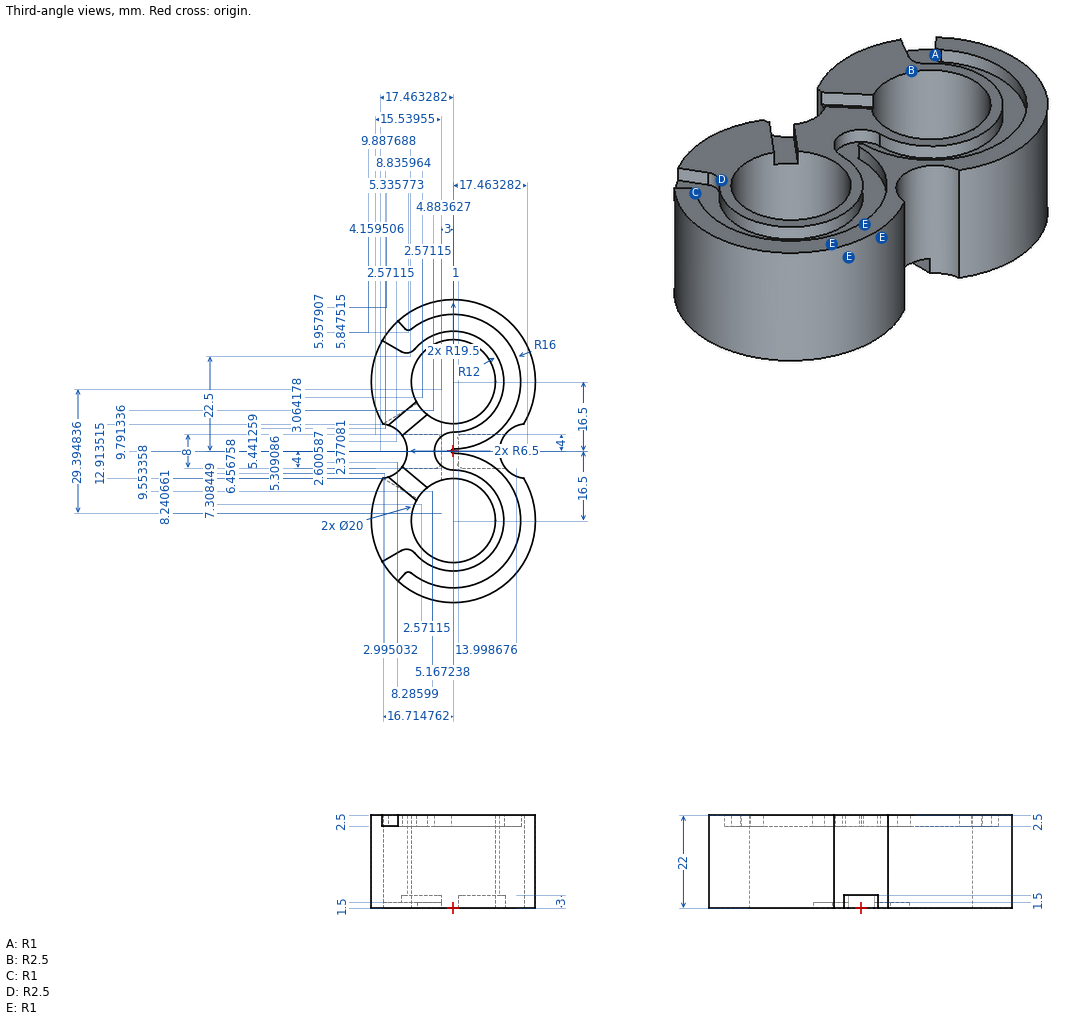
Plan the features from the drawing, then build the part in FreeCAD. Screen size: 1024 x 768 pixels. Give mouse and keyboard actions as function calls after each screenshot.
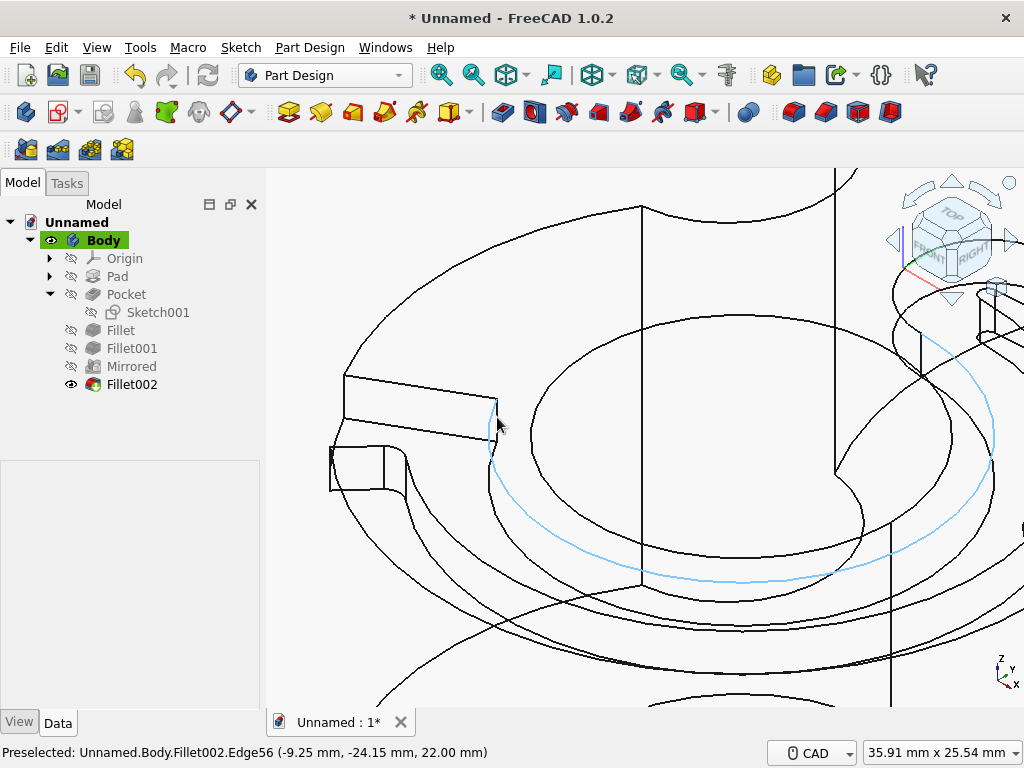
click(497, 419)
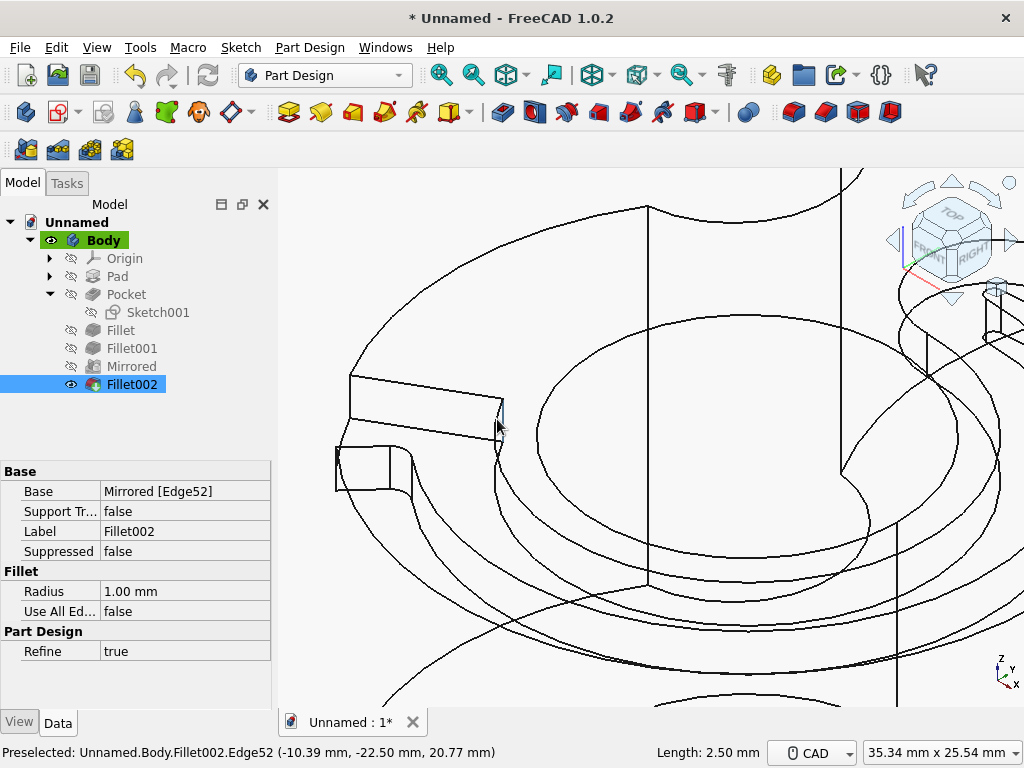
key(v)
key(1)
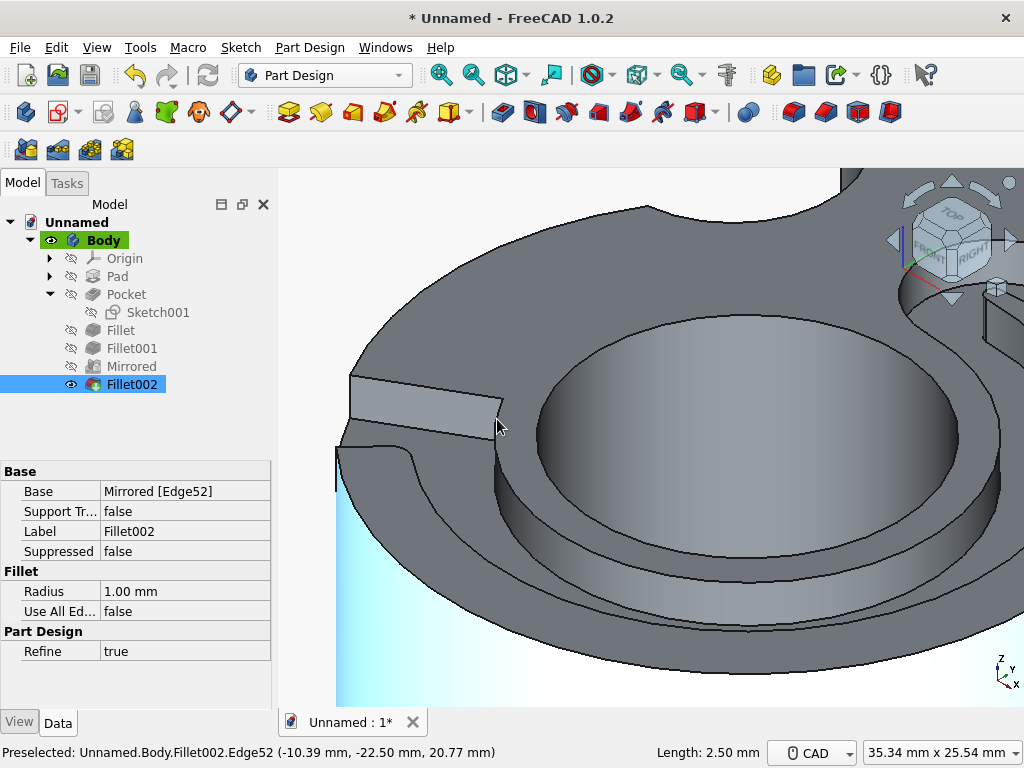
click(794, 112)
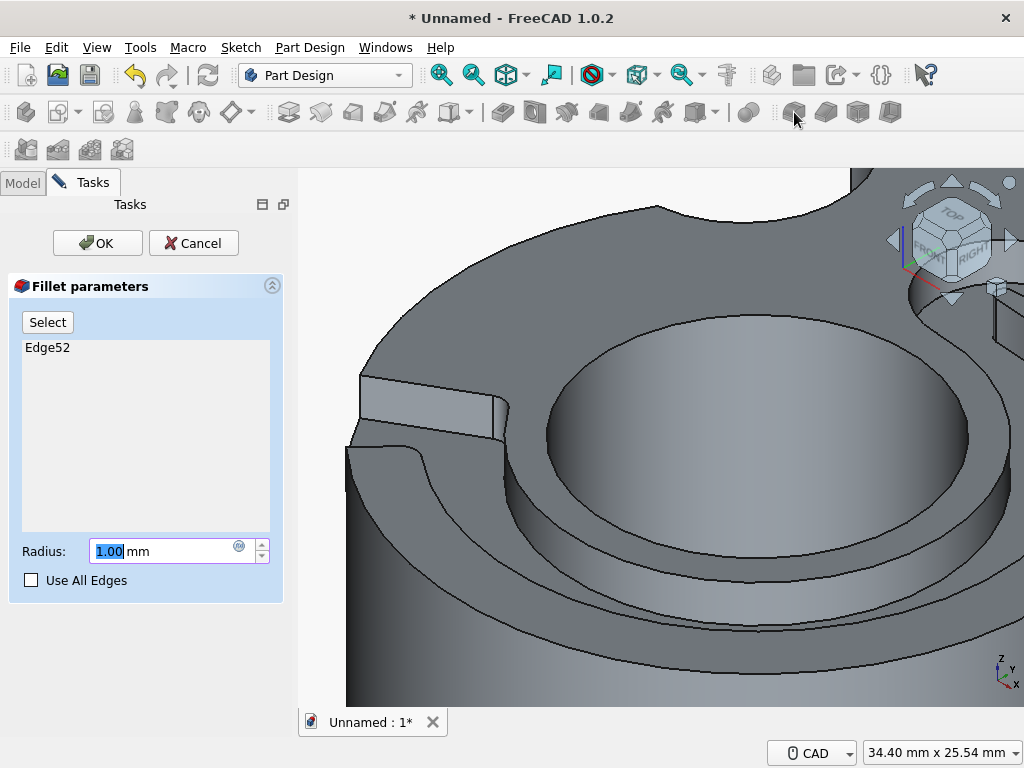
text(2.5)
key(Tab)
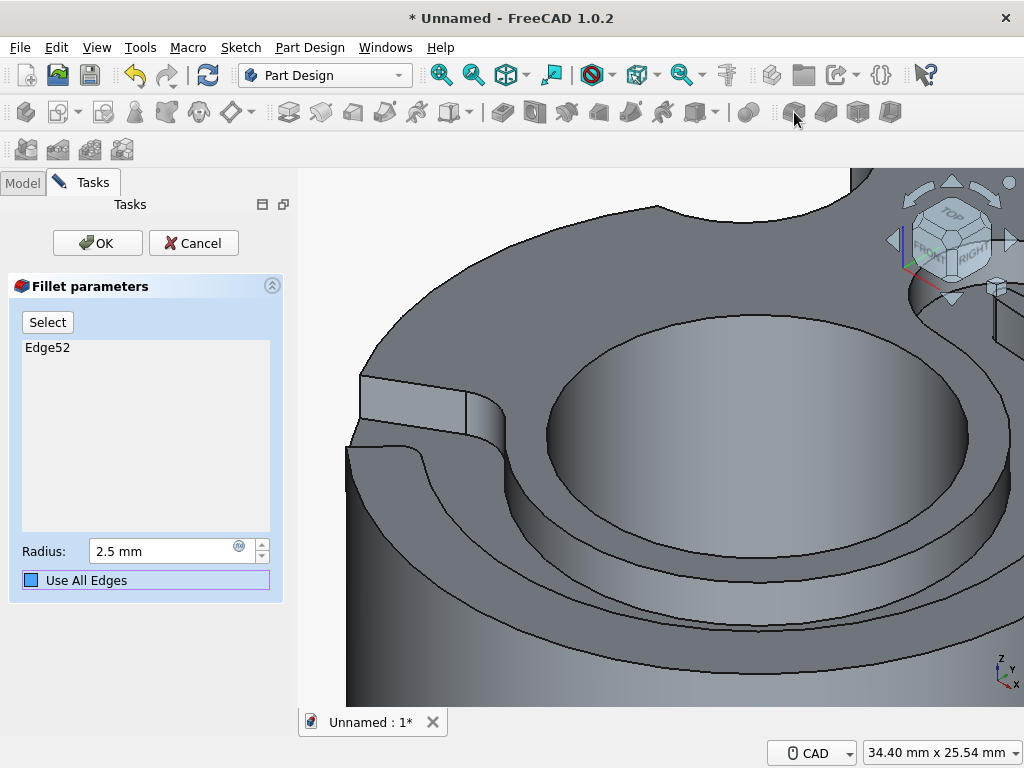
click(98, 243)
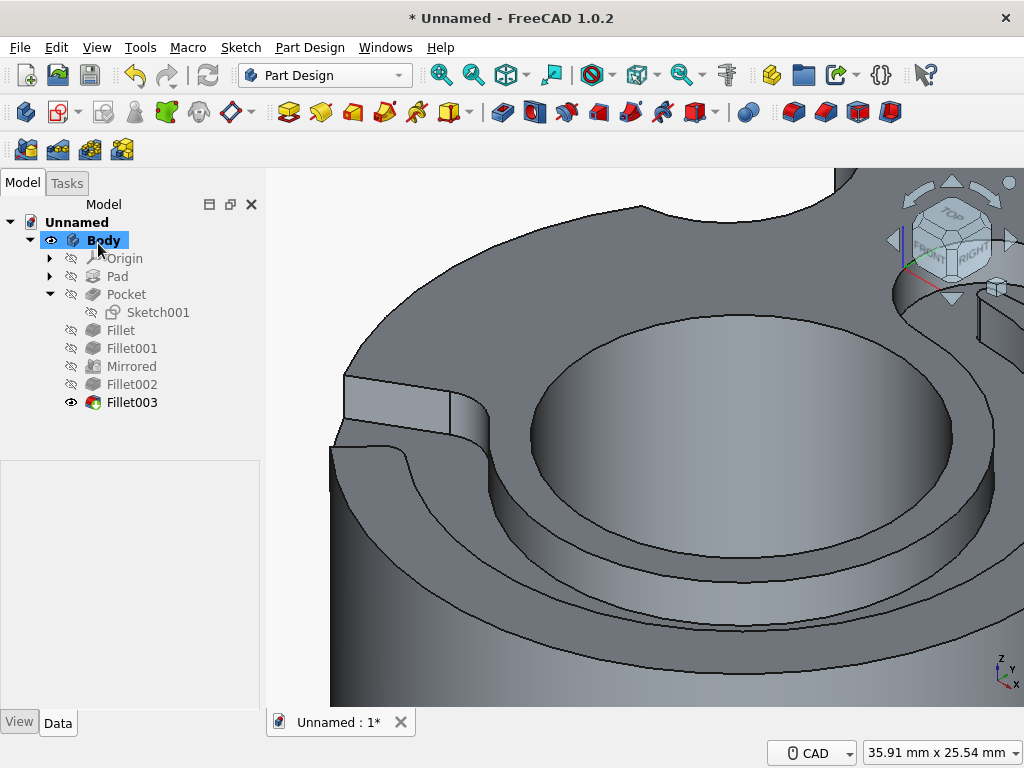
key(v)
key(f)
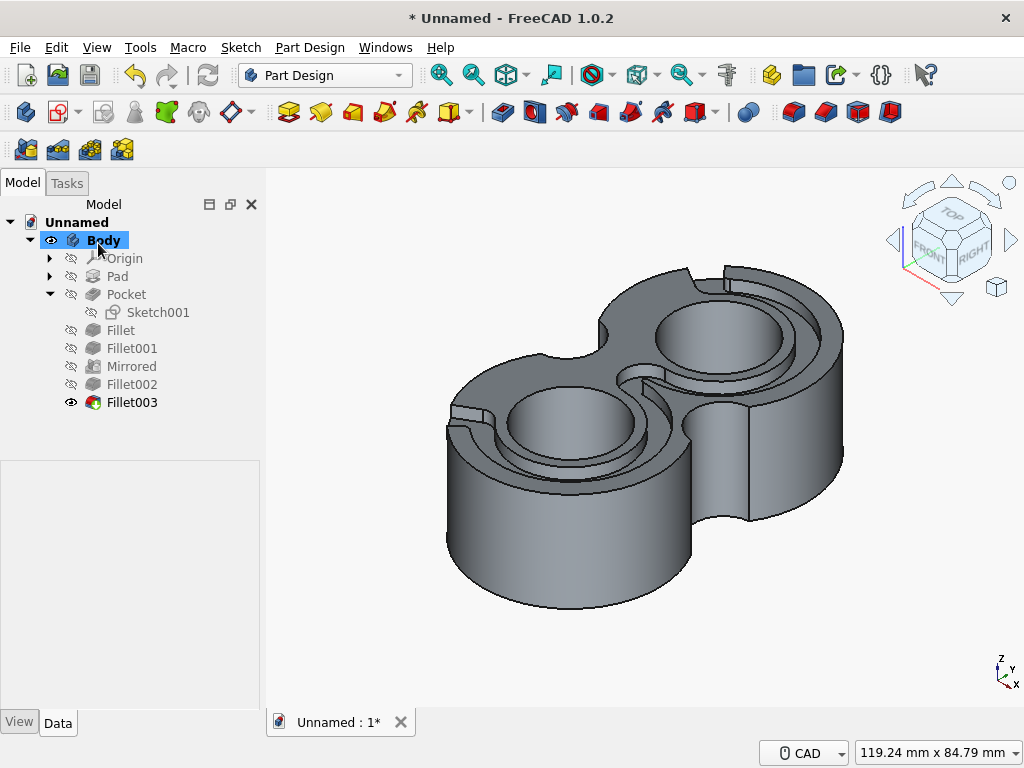
click(624, 325)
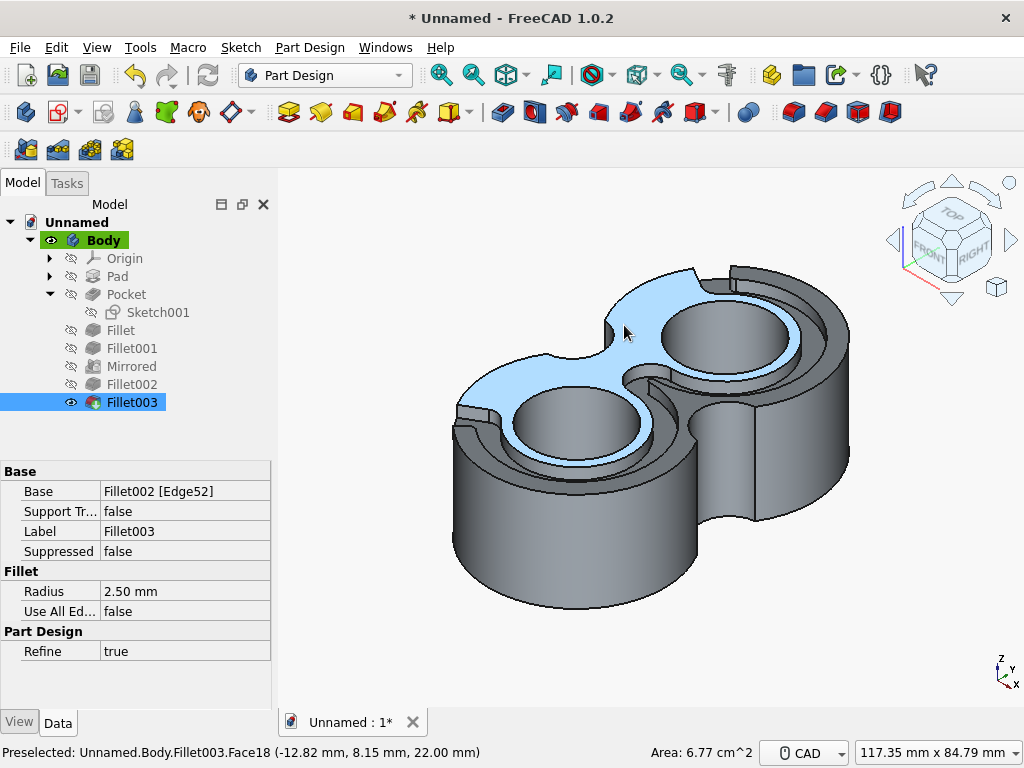
click(58, 112)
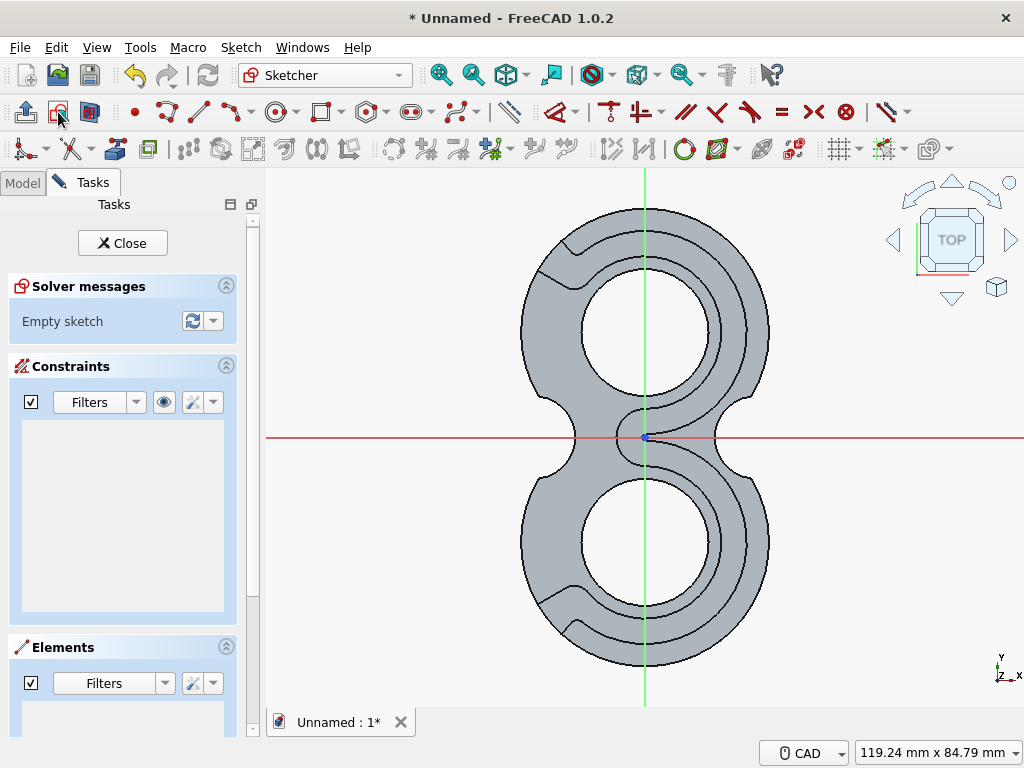
scroll(606, 436, up, 4)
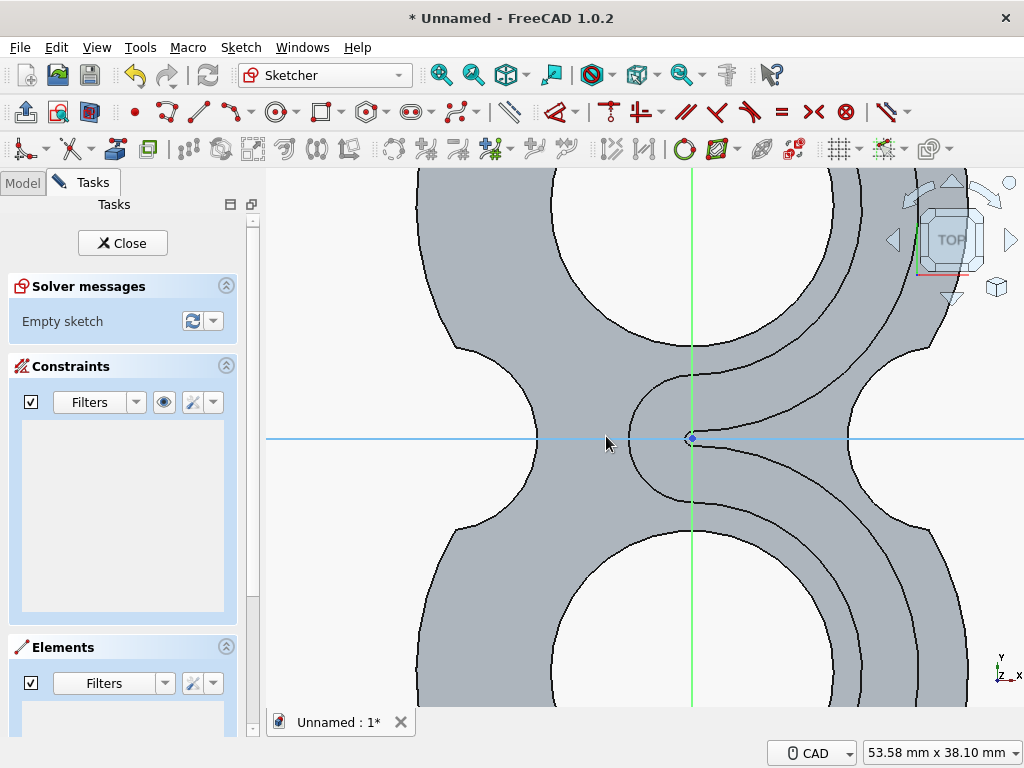
click(168, 112)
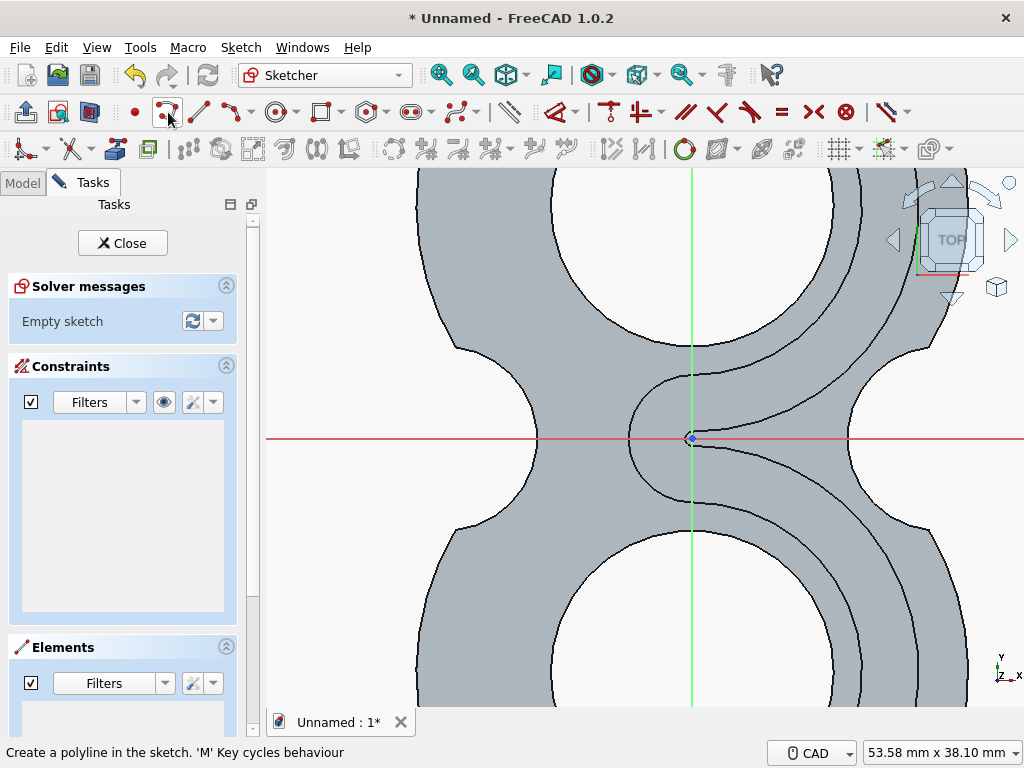
click(623, 300)
click(587, 257)
click(462, 362)
click(498, 405)
click(623, 301)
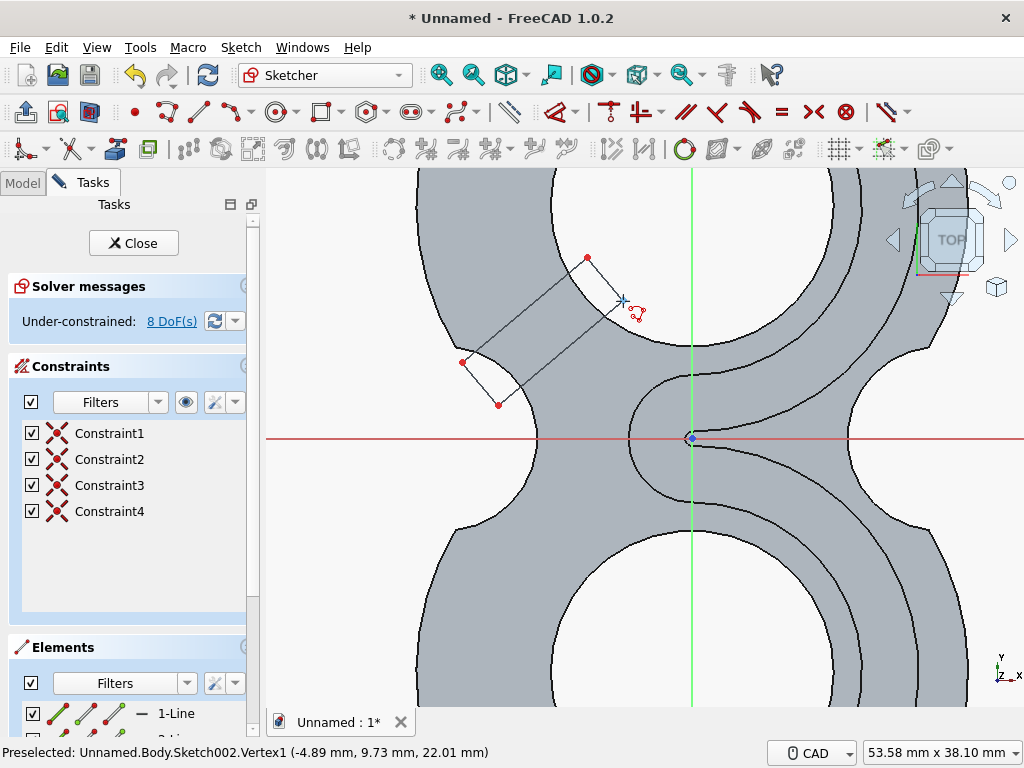
click(619, 574)
click(502, 476)
click(460, 514)
click(583, 617)
click(619, 575)
key(Escape)
key(Escape)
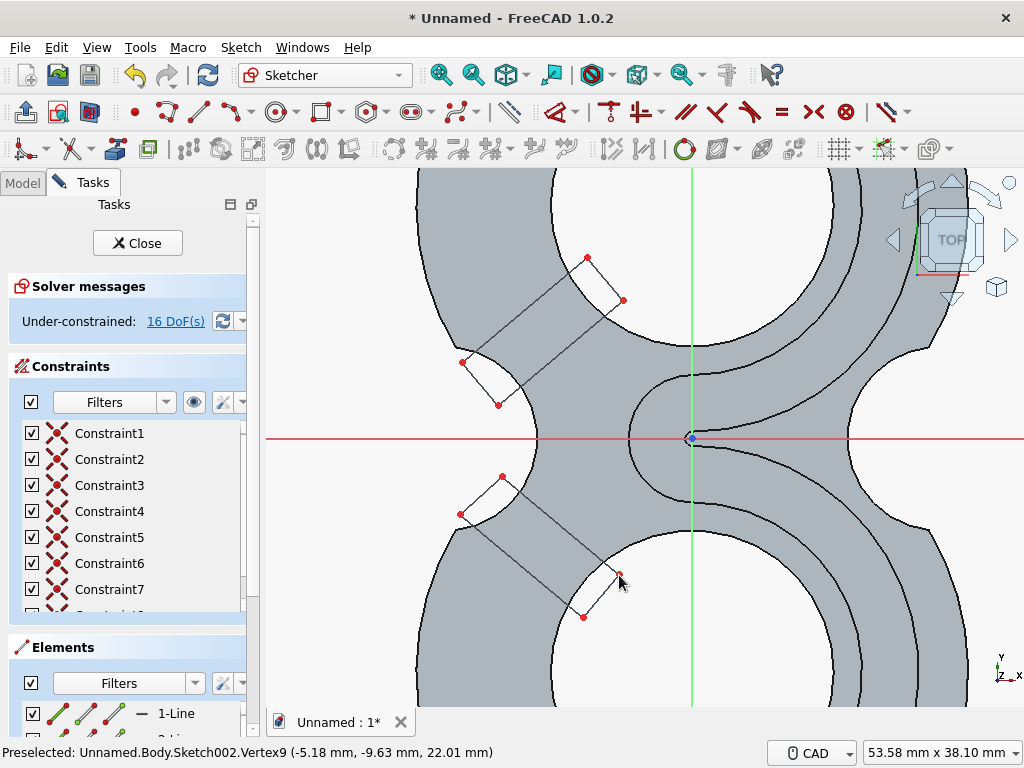
click(612, 288)